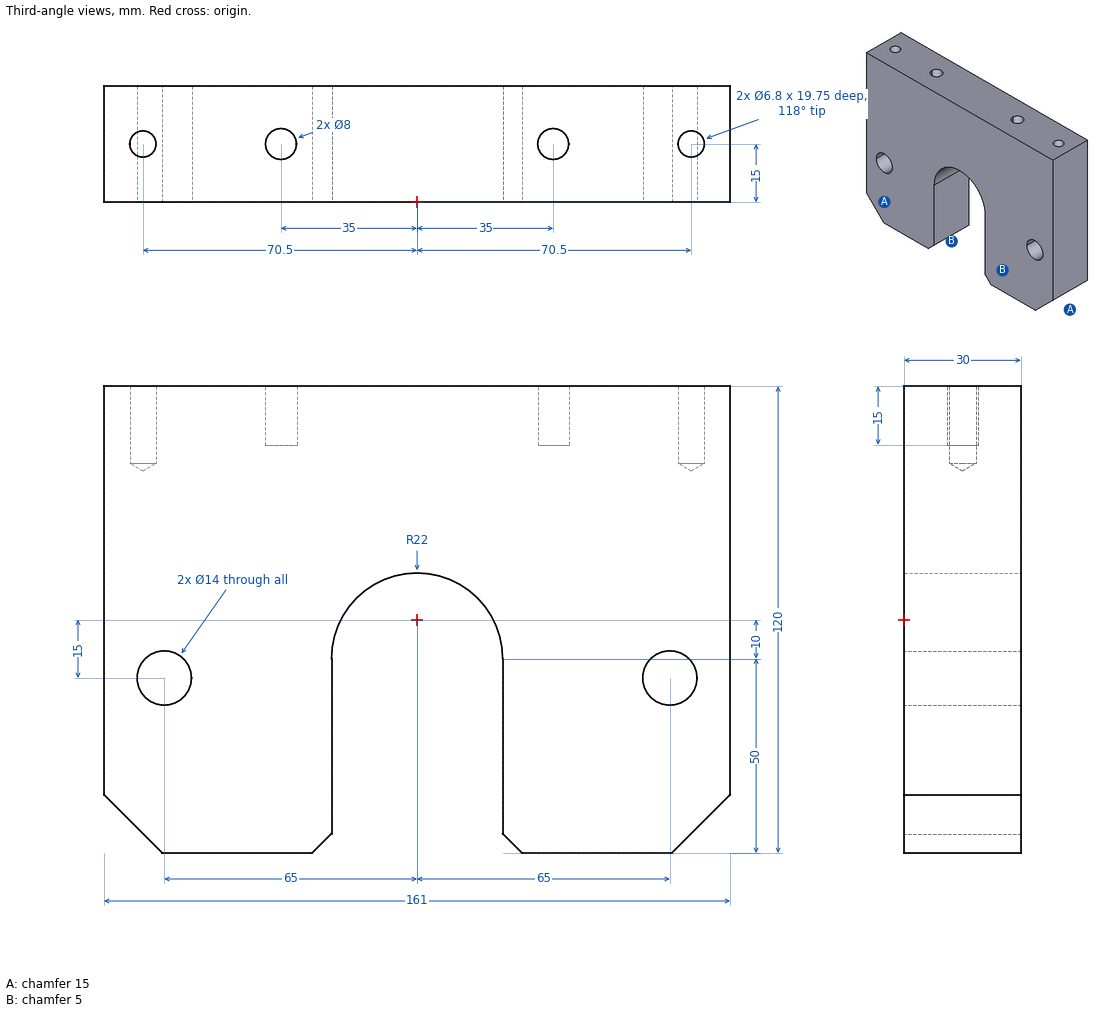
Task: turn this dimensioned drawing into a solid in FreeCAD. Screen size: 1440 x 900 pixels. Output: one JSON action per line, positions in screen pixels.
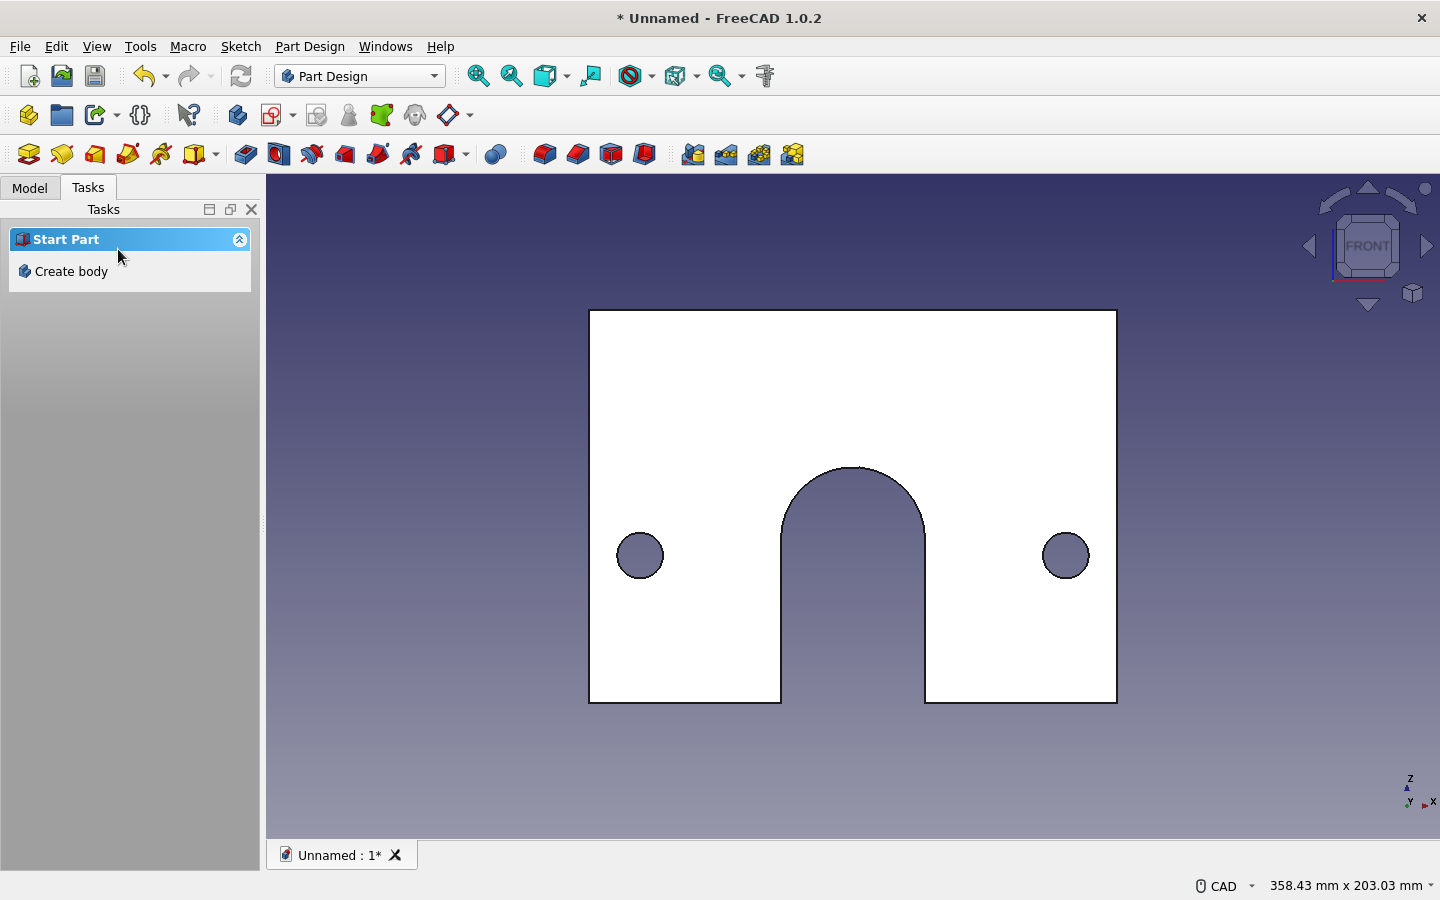
{"action": "key", "text": "3"}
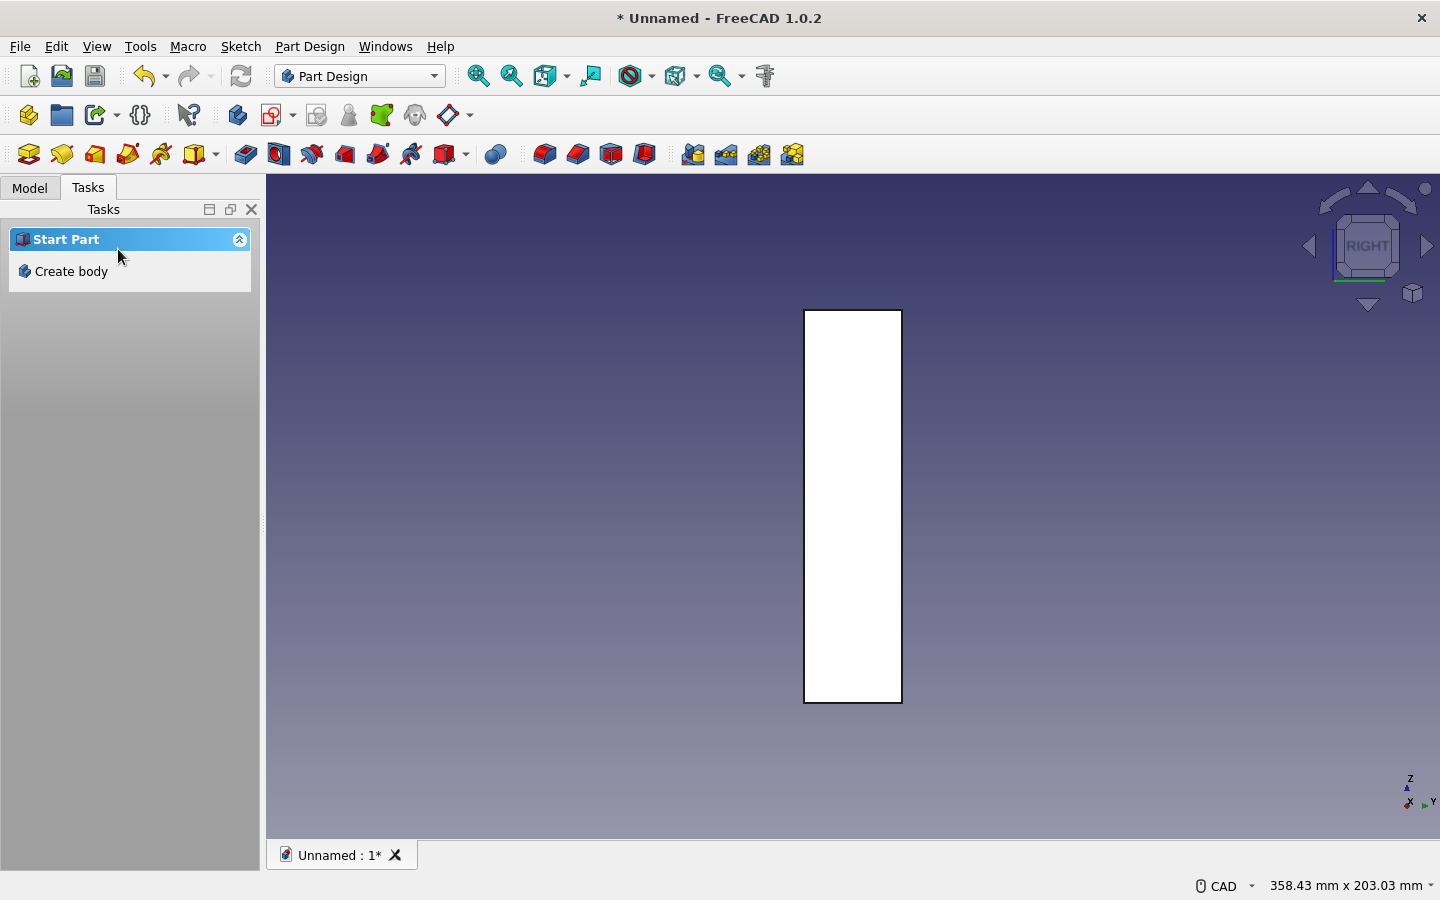
{"action": "left_click", "coordinate": [853, 702]}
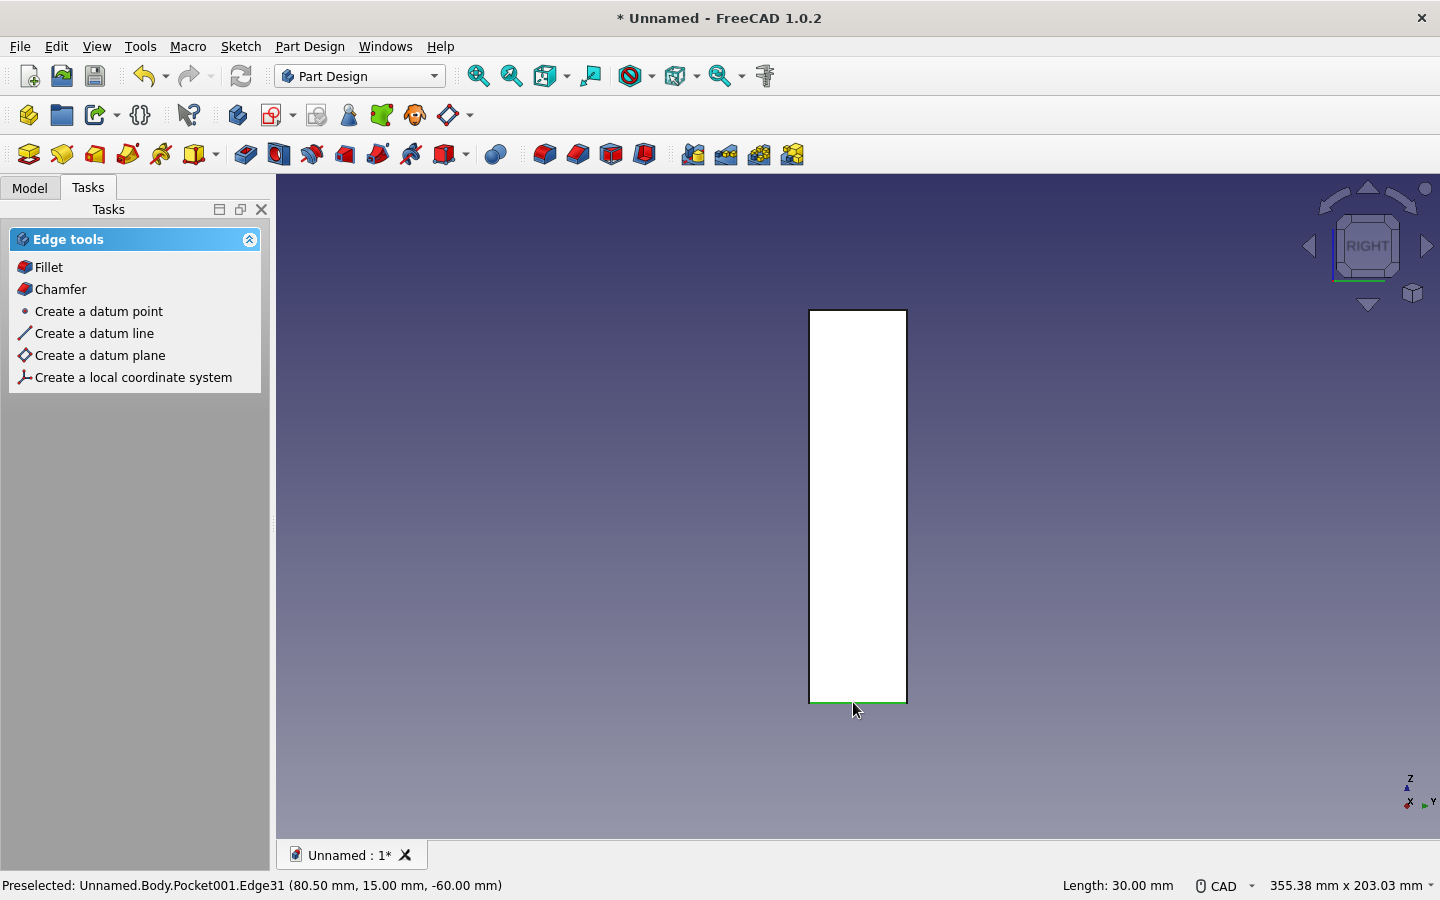
{"action": "key", "text": "5"}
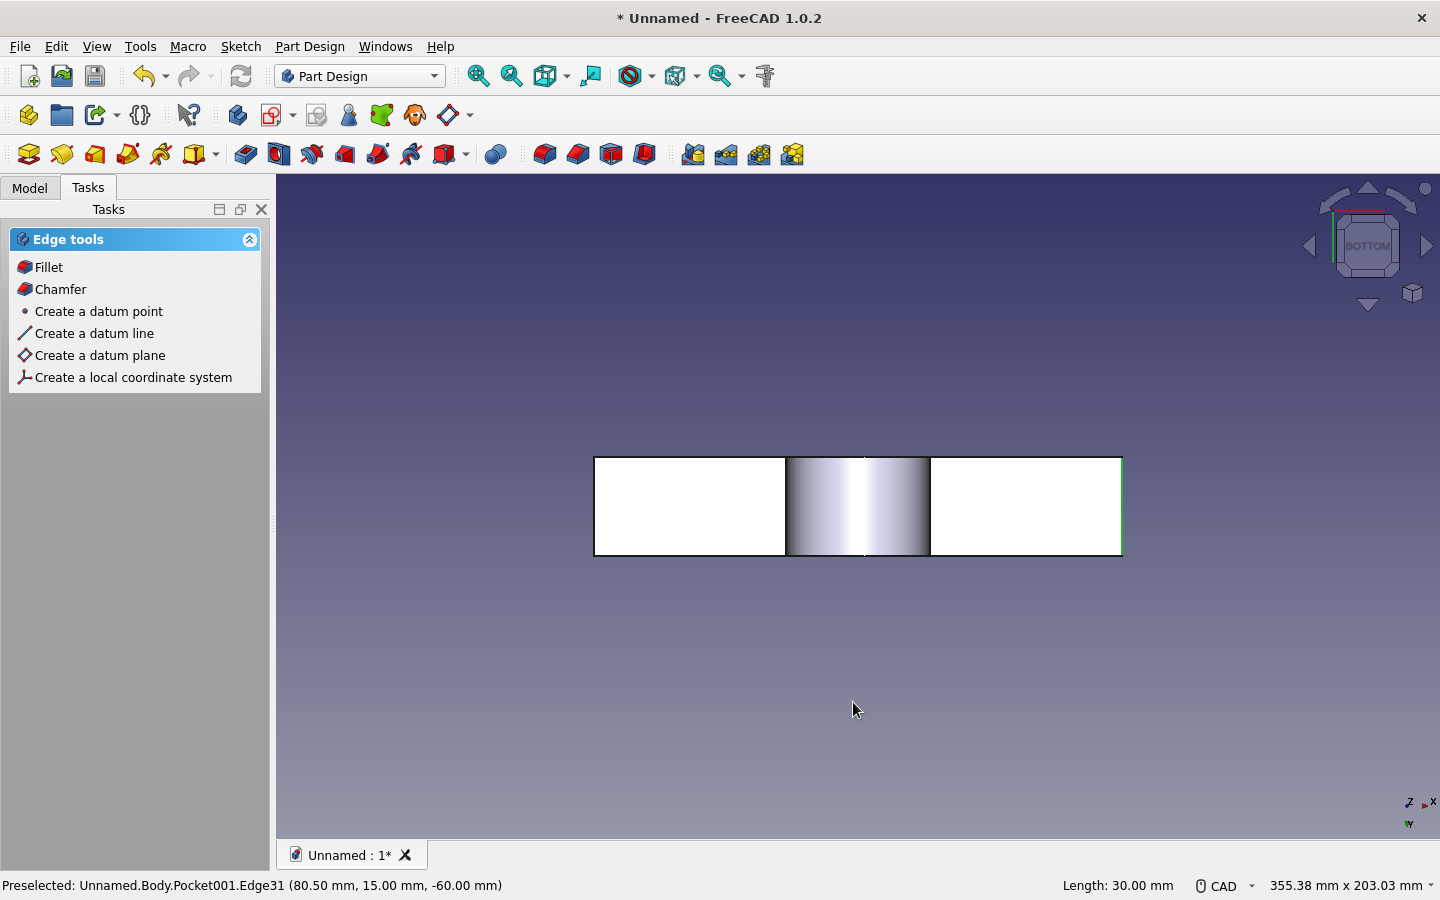
{"action": "left_click", "coordinate": [594, 505], "text": "ctrl"}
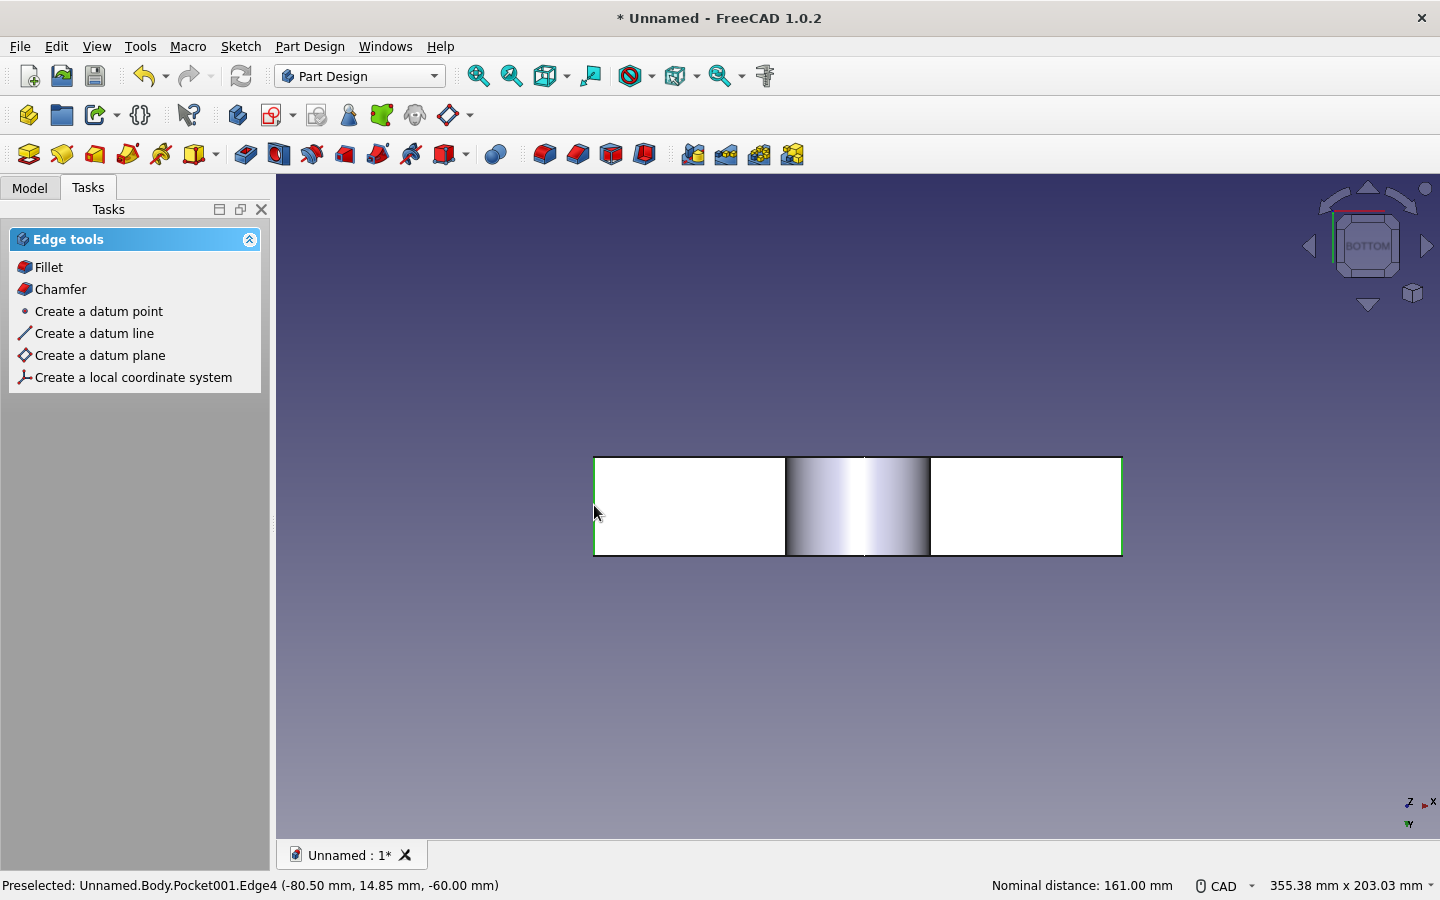
{"action": "left_click", "coordinate": [578, 154]}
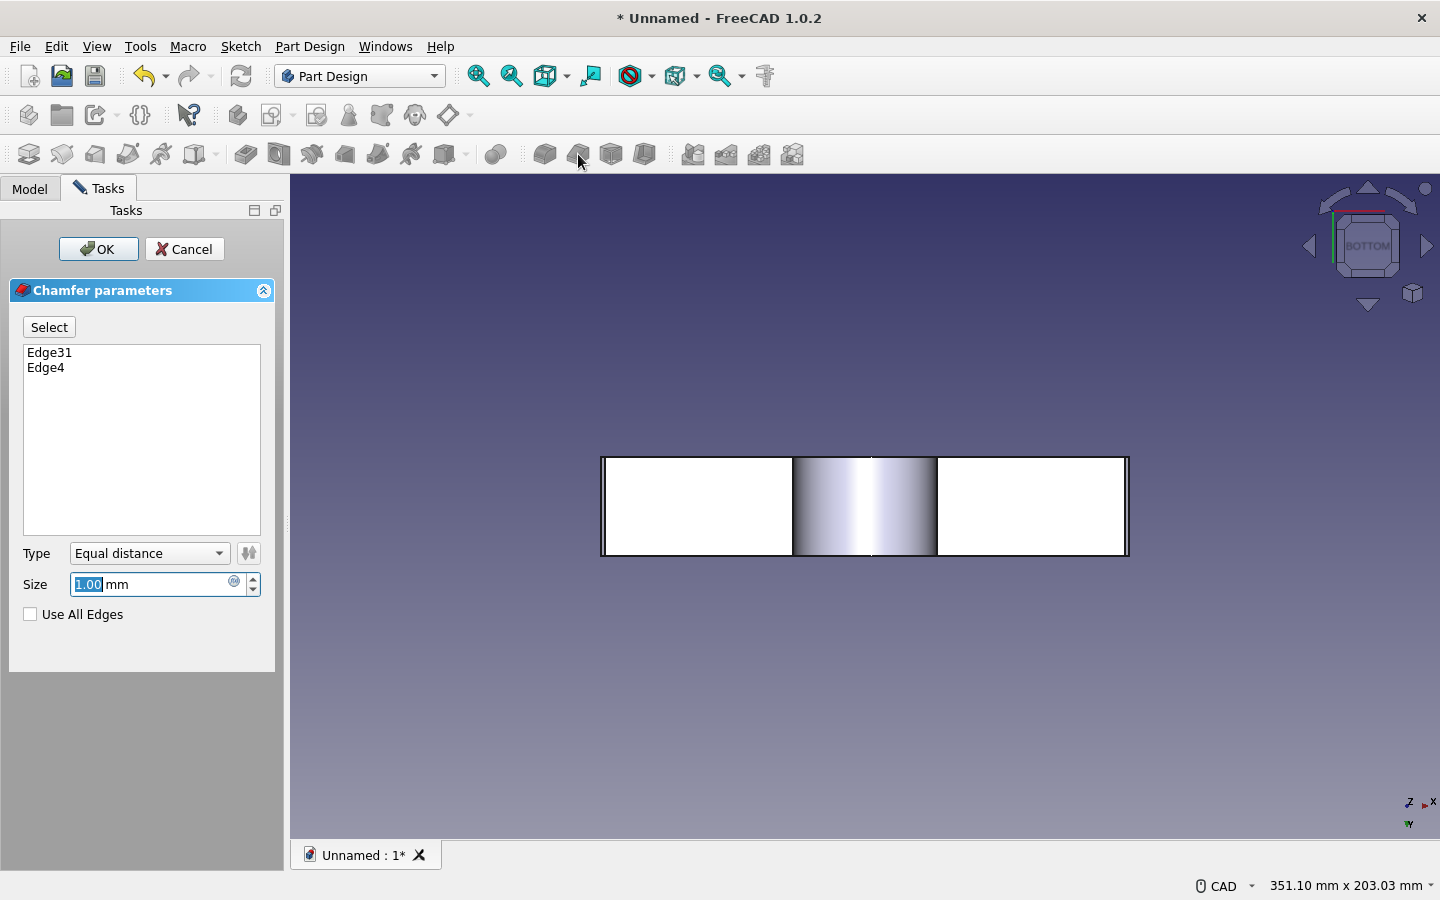
{"action": "type", "text": "15"}
{"action": "key", "text": "Tab"}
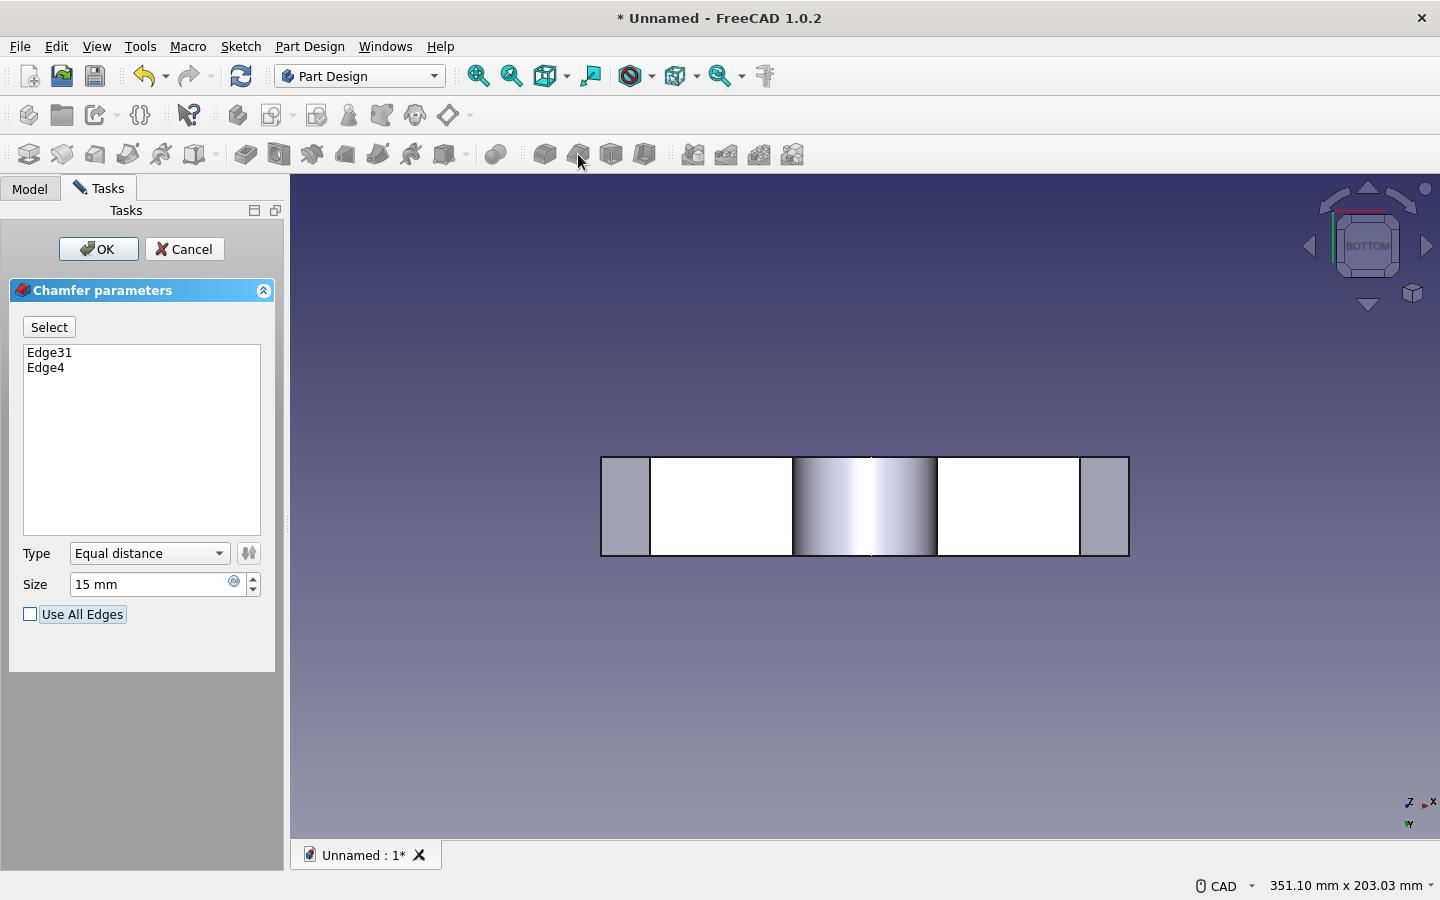
{"action": "left_click", "coordinate": [99, 249]}